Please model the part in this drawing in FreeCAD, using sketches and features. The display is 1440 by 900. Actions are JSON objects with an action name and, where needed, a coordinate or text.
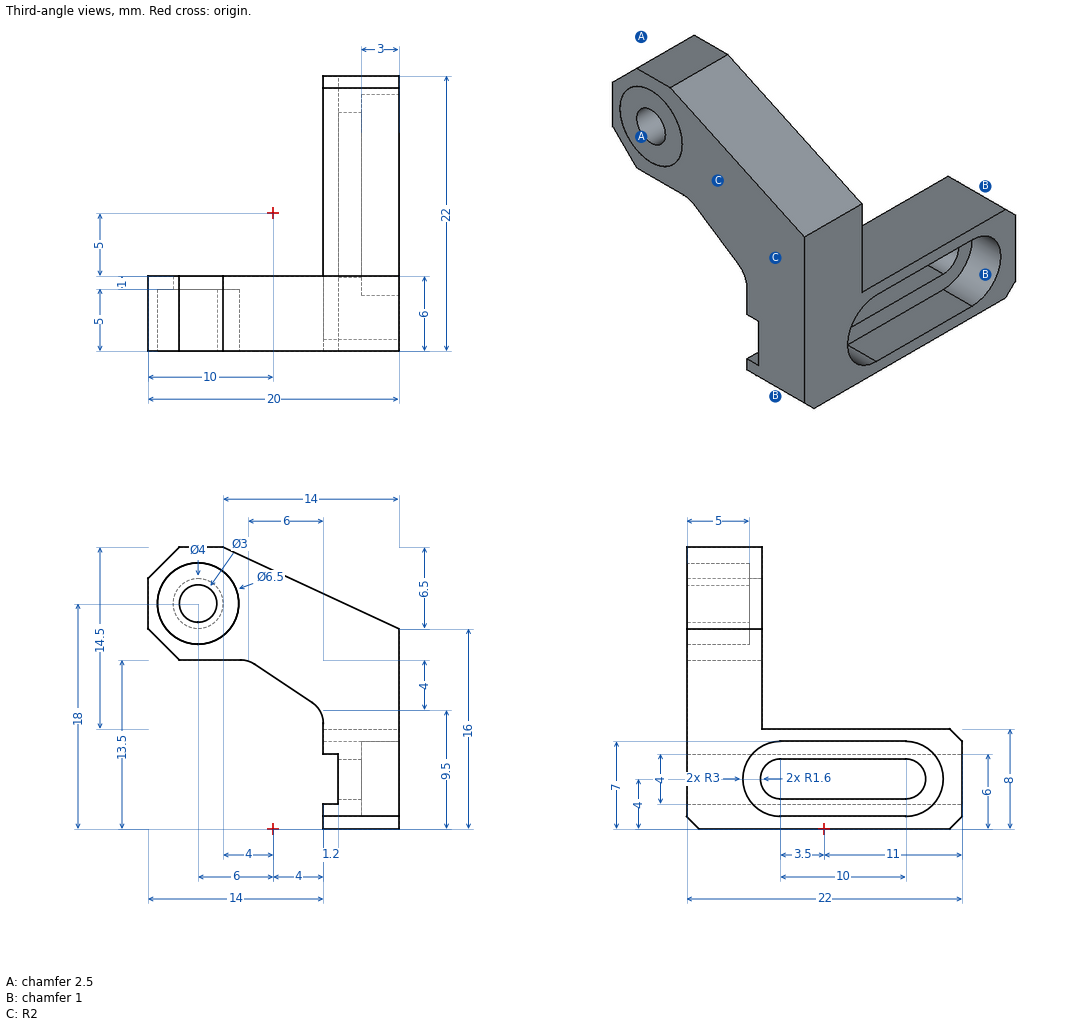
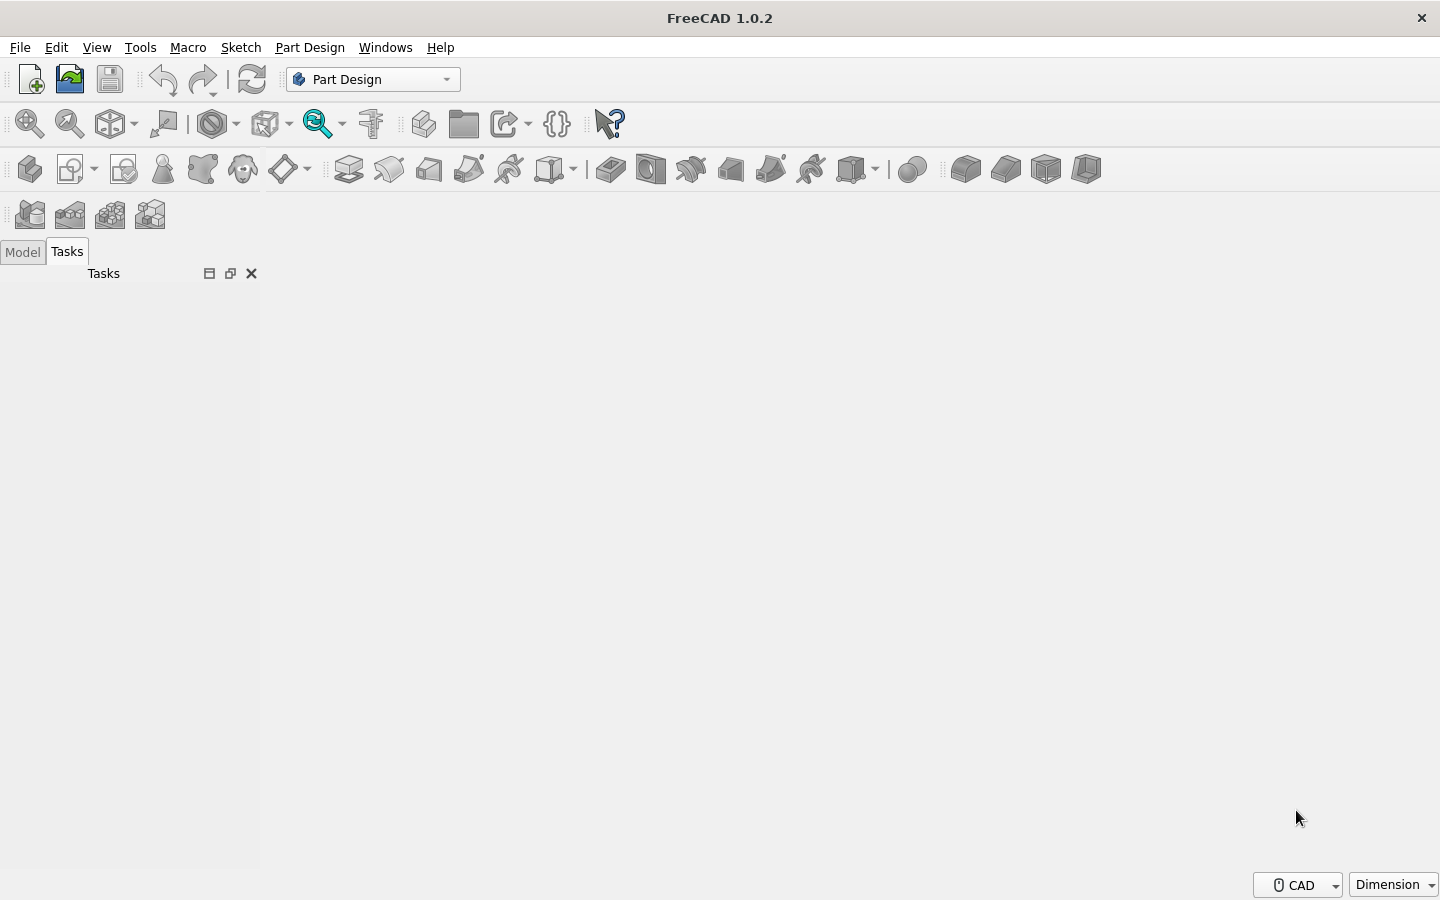
{"action": "left_click", "coordinate": [916, 124]}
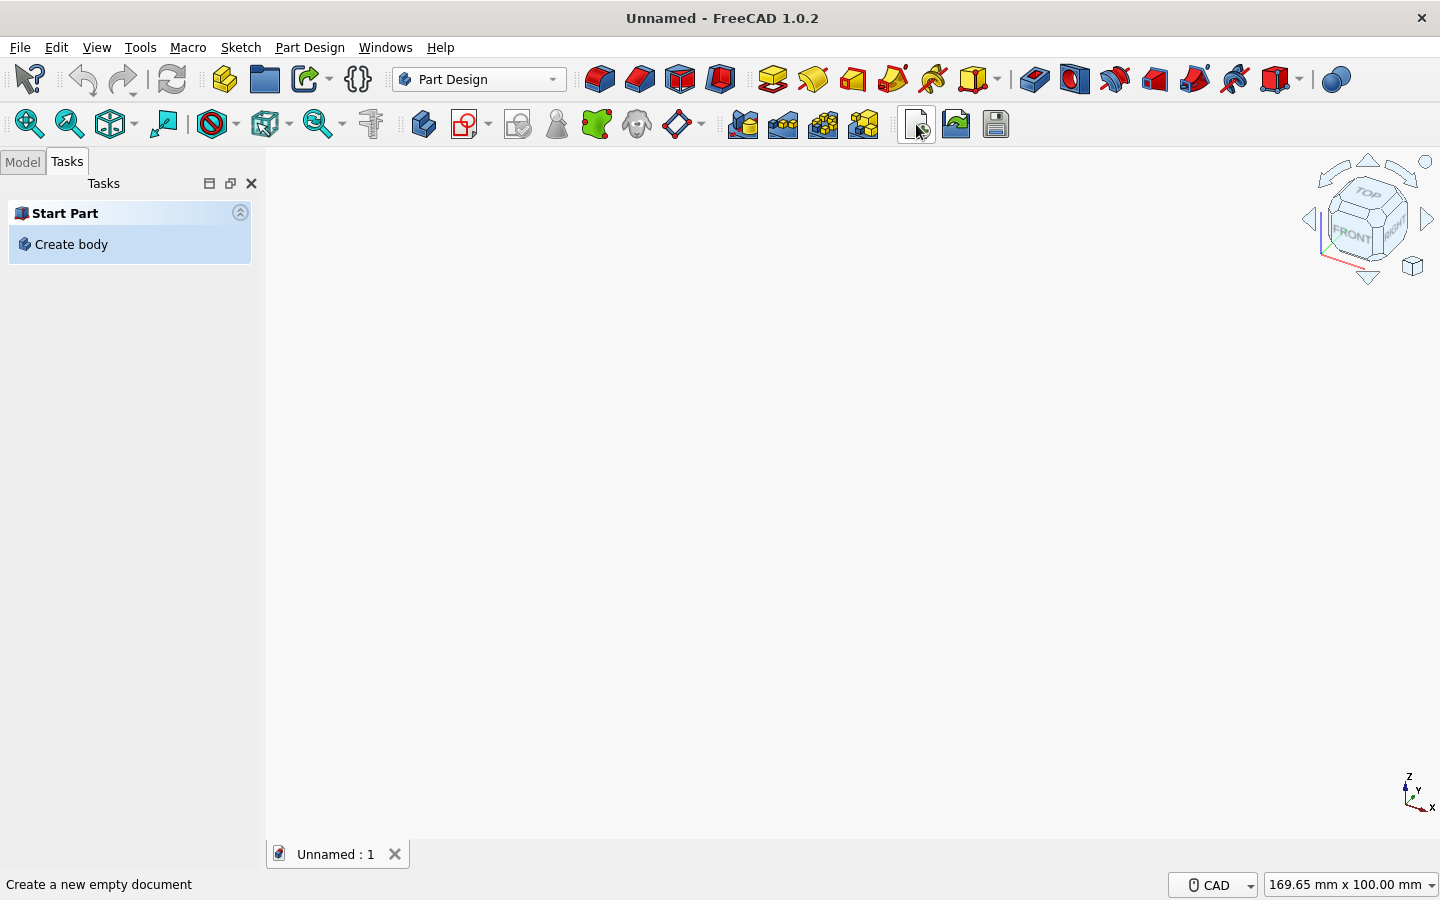
{"action": "left_click", "coordinate": [464, 124]}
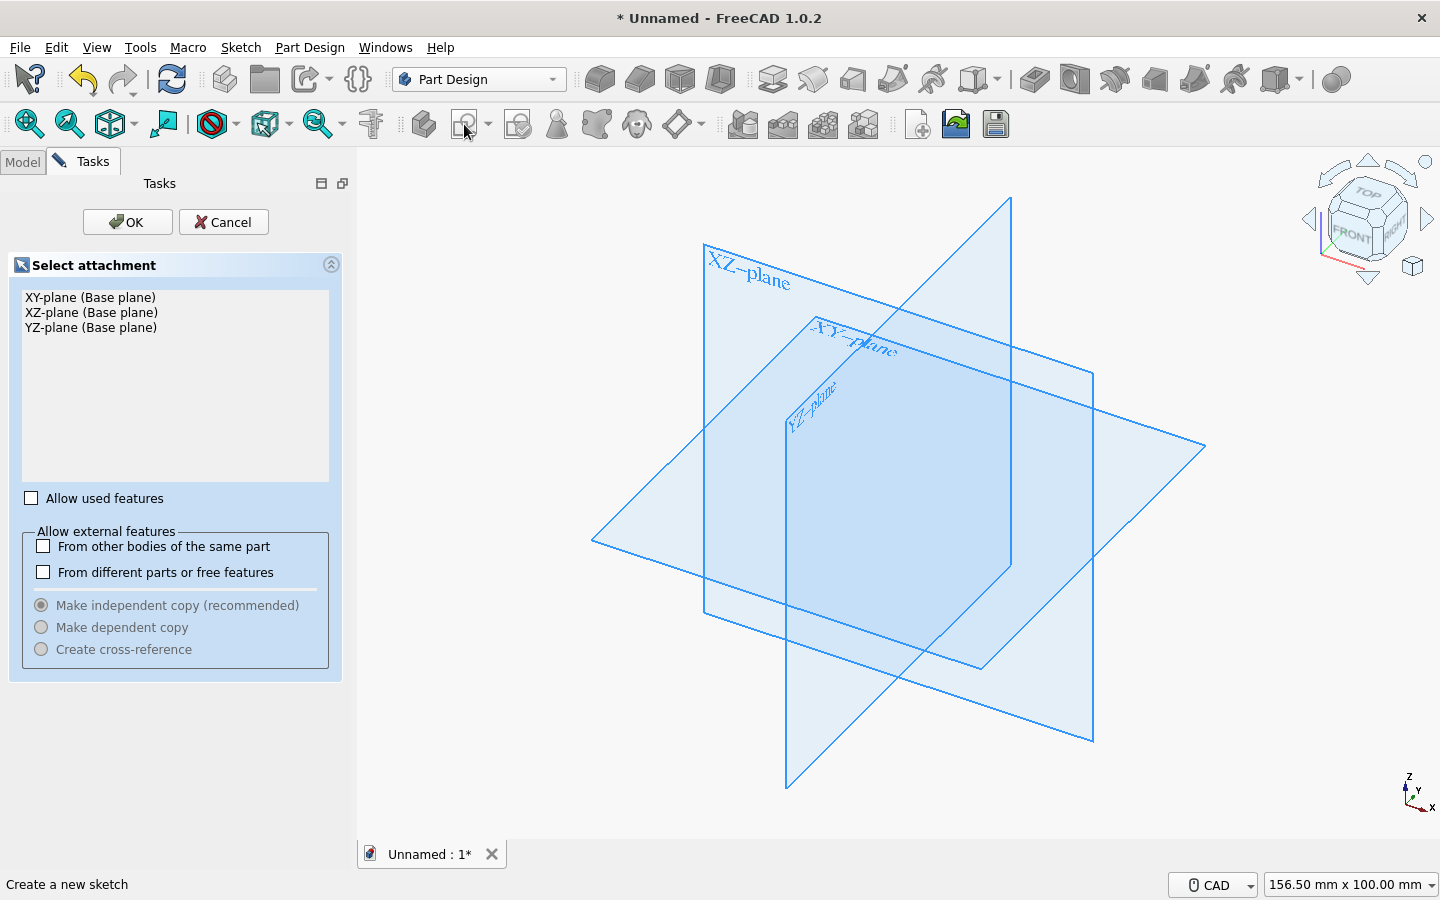
{"action": "left_click", "coordinate": [82, 298]}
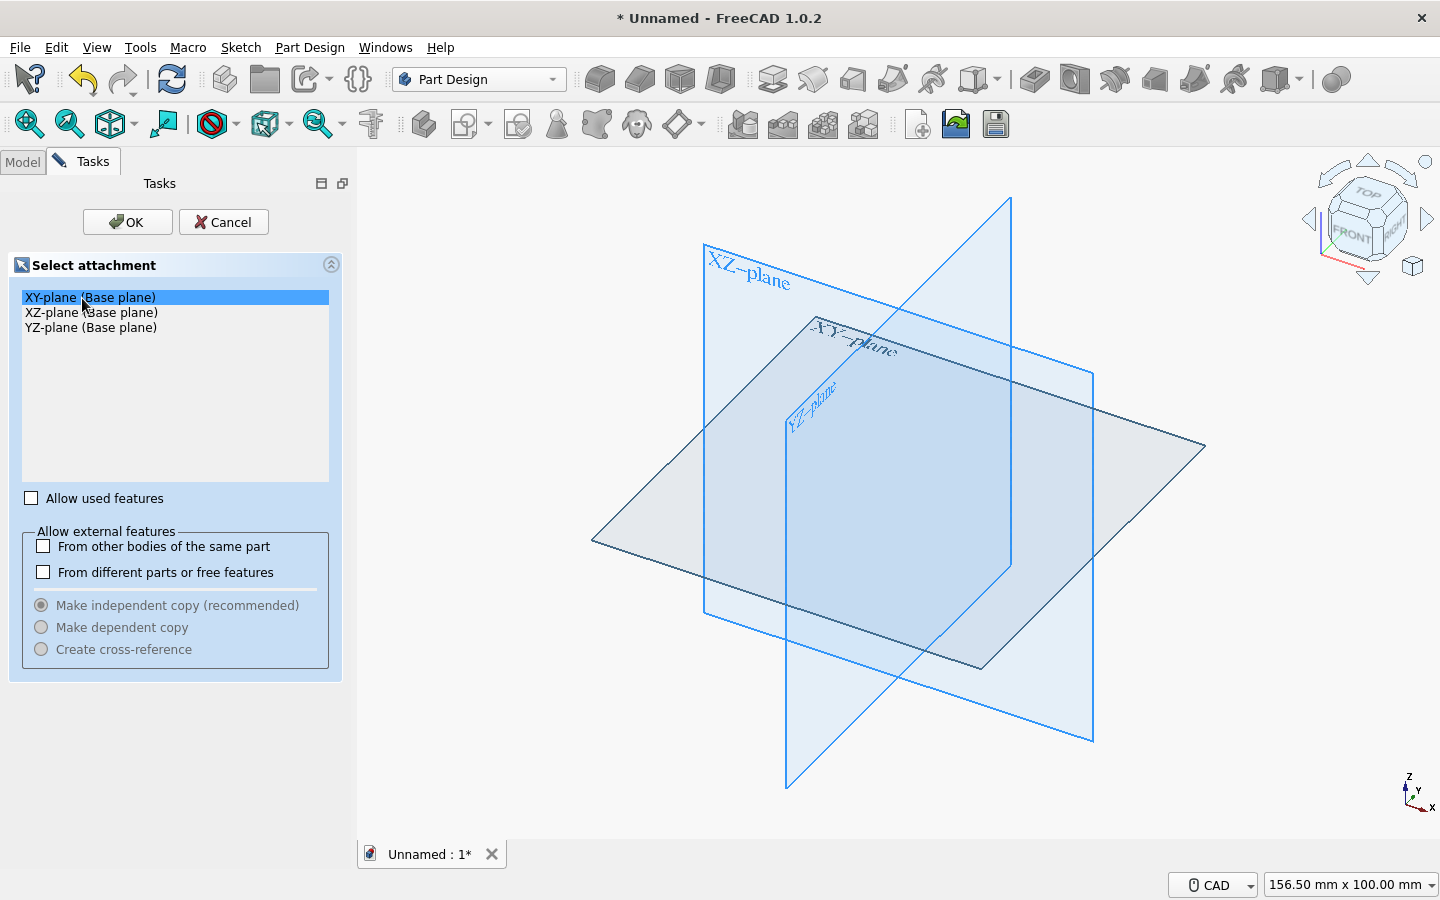
{"action": "left_click", "coordinate": [128, 222]}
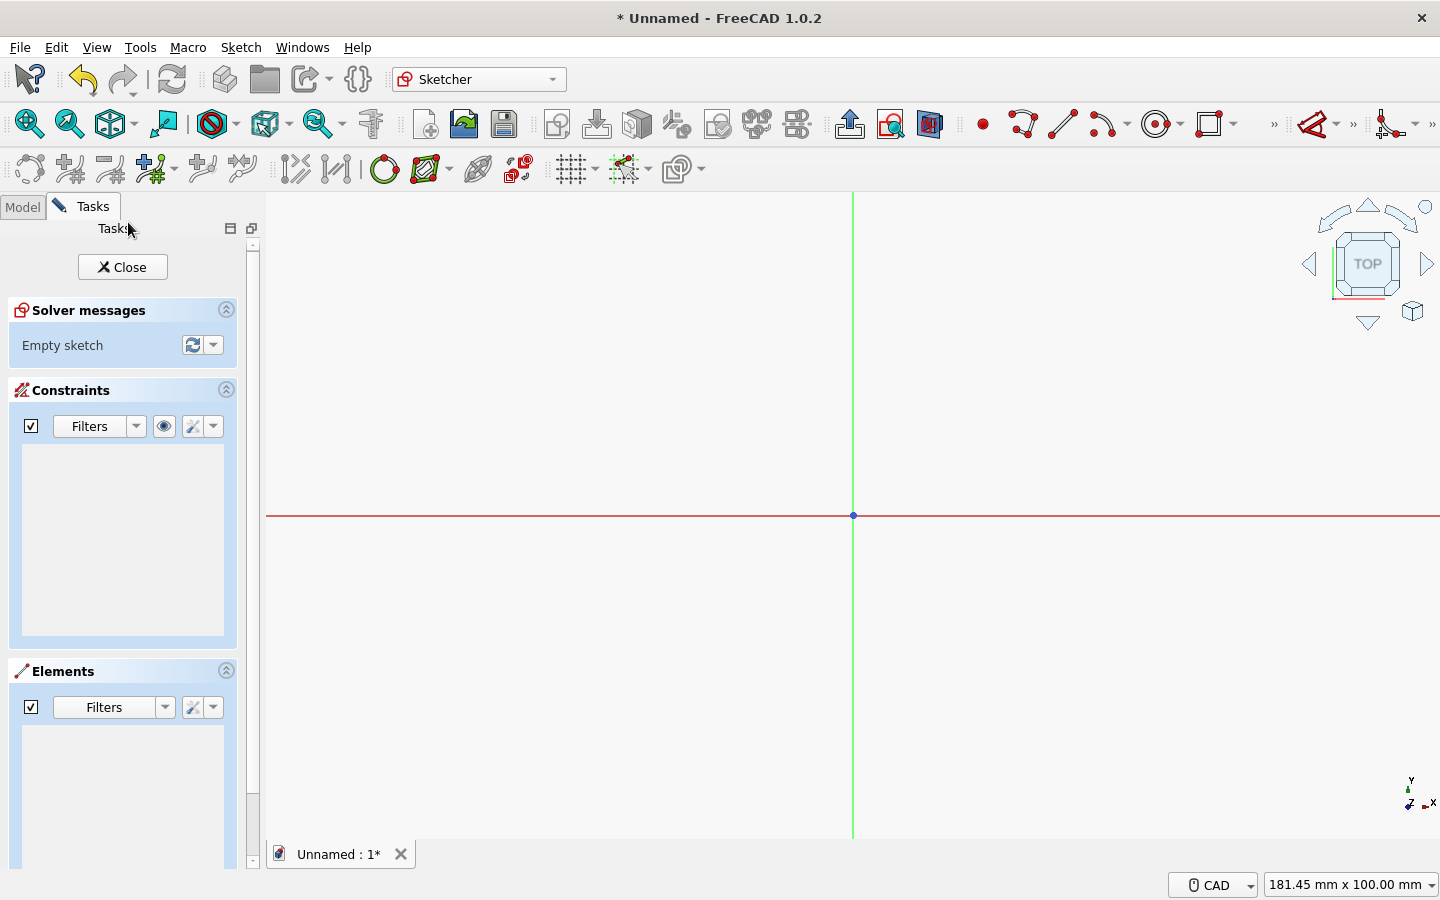
{"action": "scroll", "coordinate": [893, 516], "scroll_direction": "up", "scroll_amount": 5}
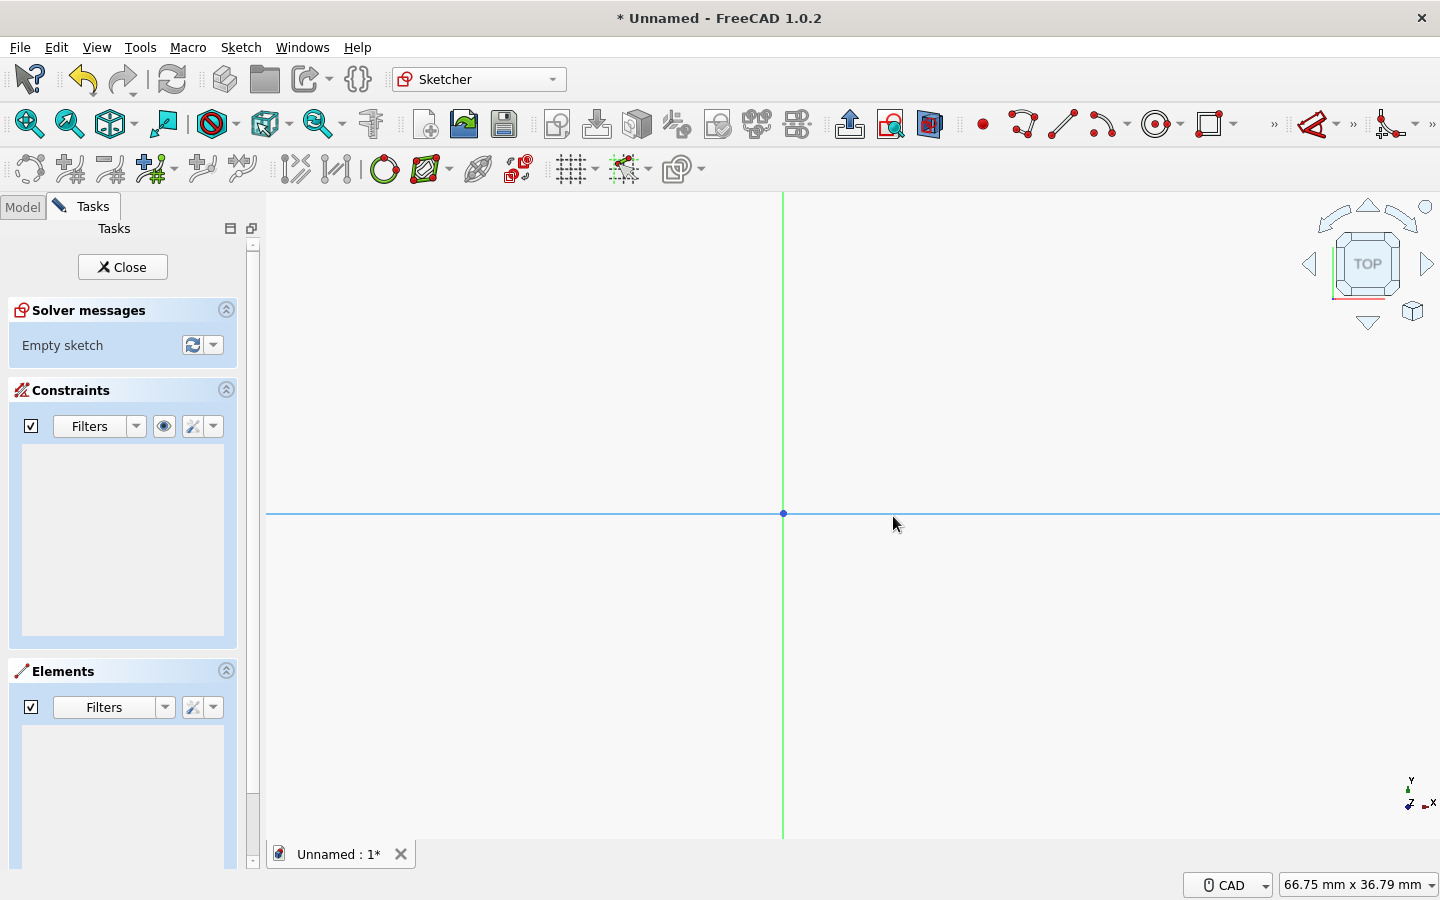
{"action": "left_click", "coordinate": [1236, 124]}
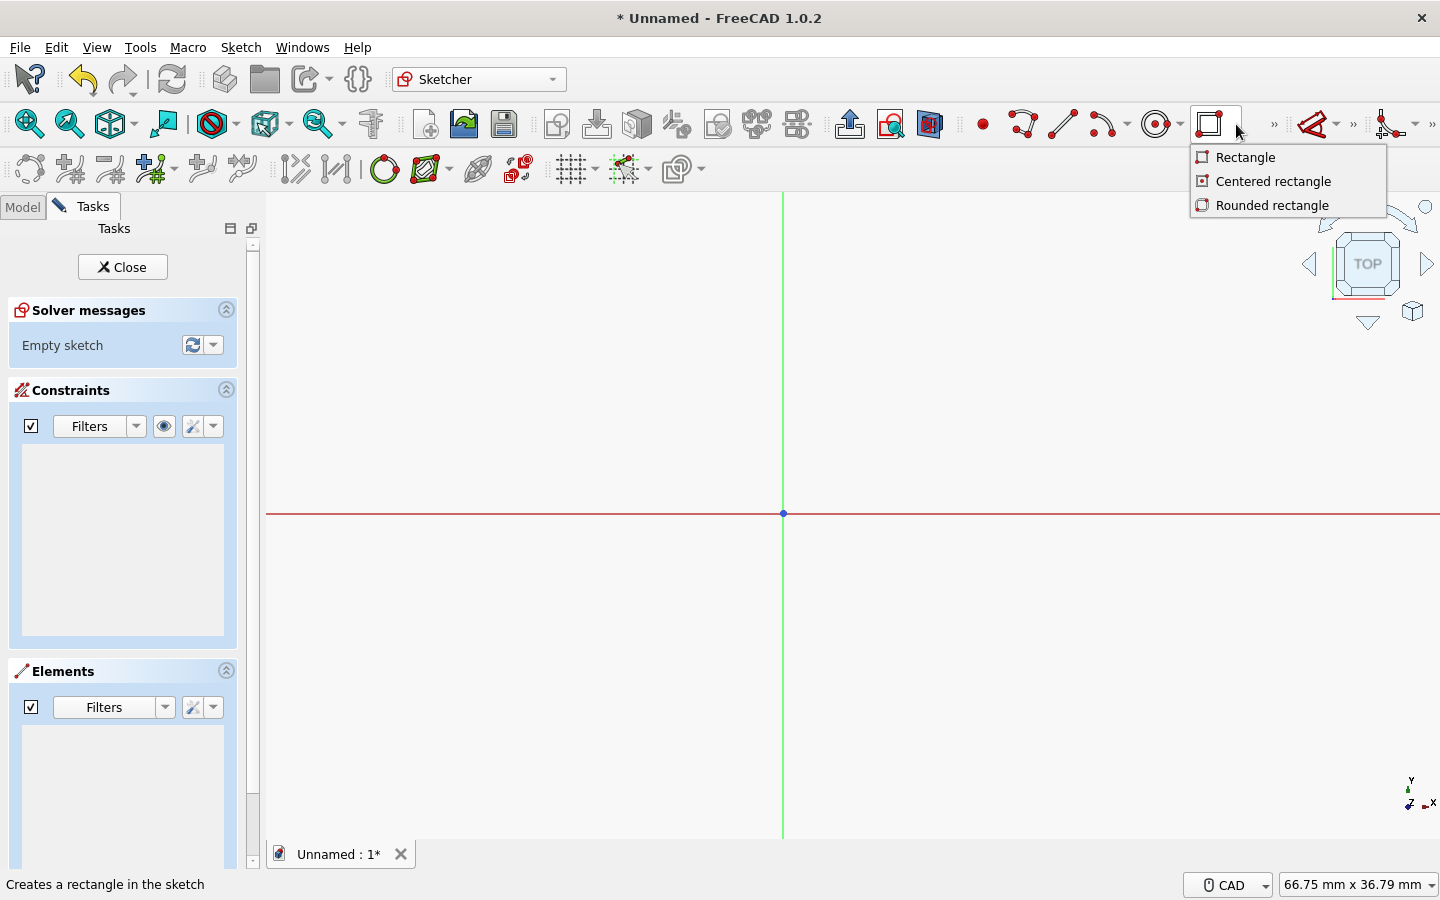
{"action": "left_click", "coordinate": [1288, 181]}